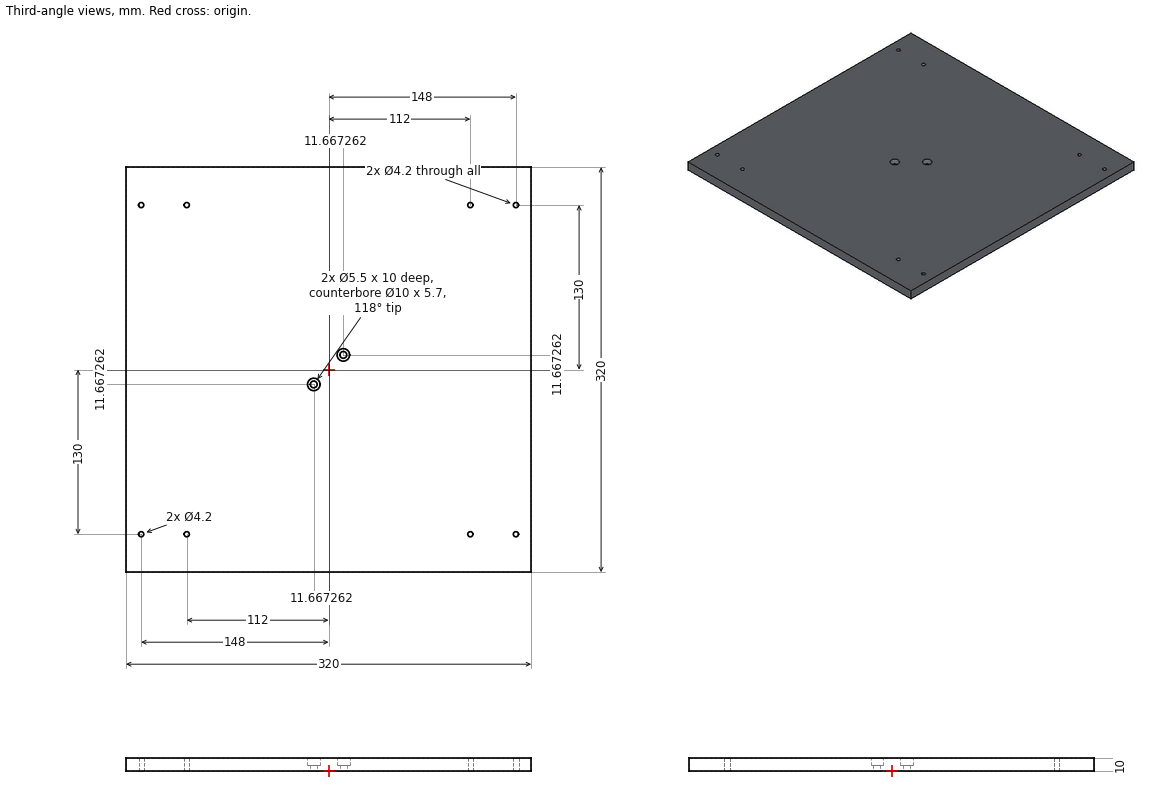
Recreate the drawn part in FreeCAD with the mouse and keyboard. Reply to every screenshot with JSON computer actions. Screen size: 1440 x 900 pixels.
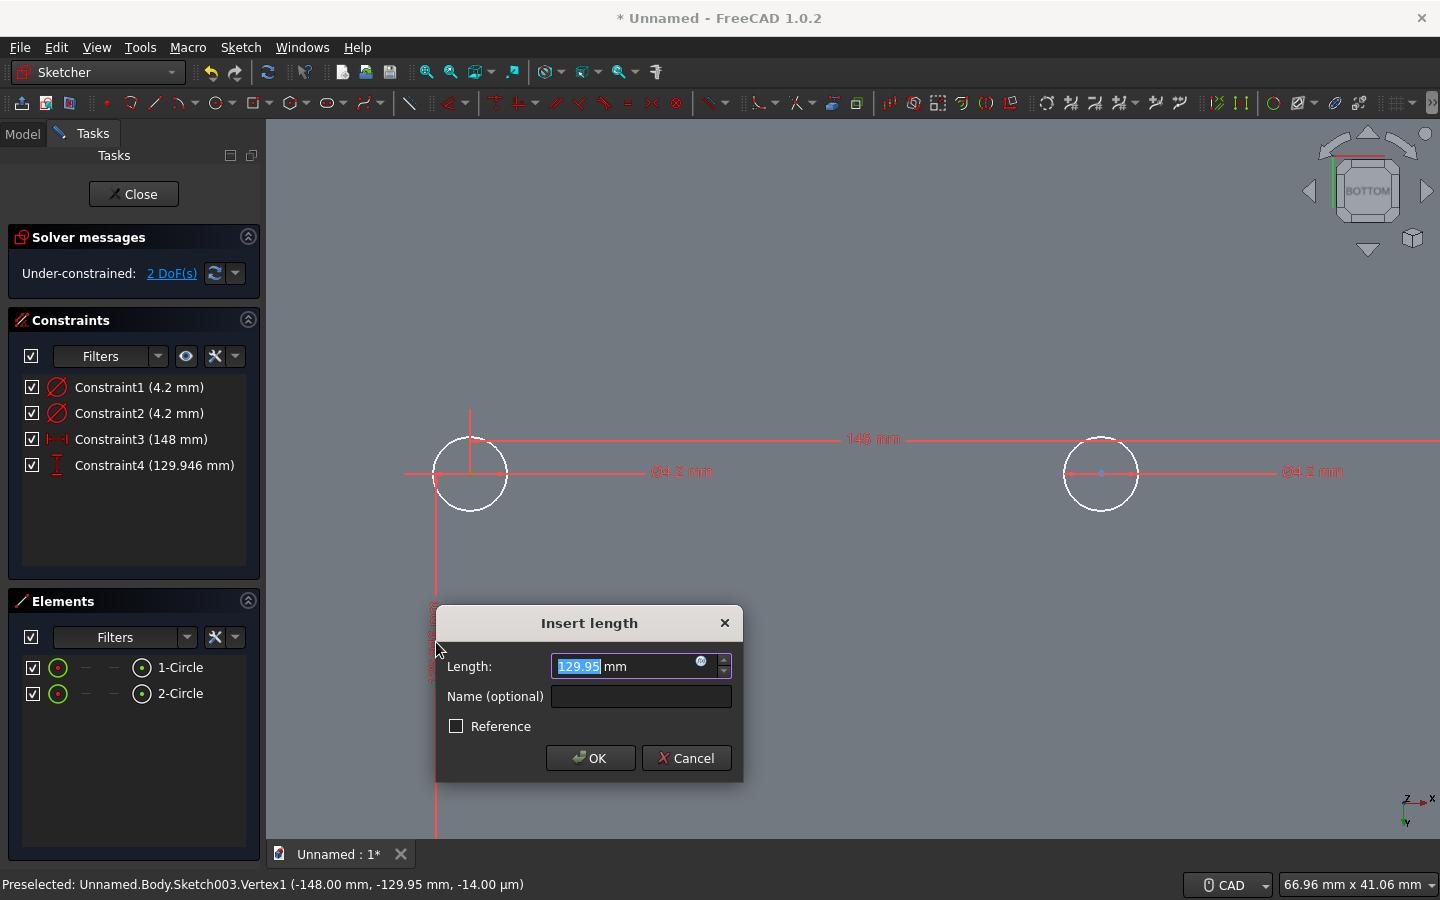
{"action": "type", "text": "130"}
{"action": "key", "text": "Return"}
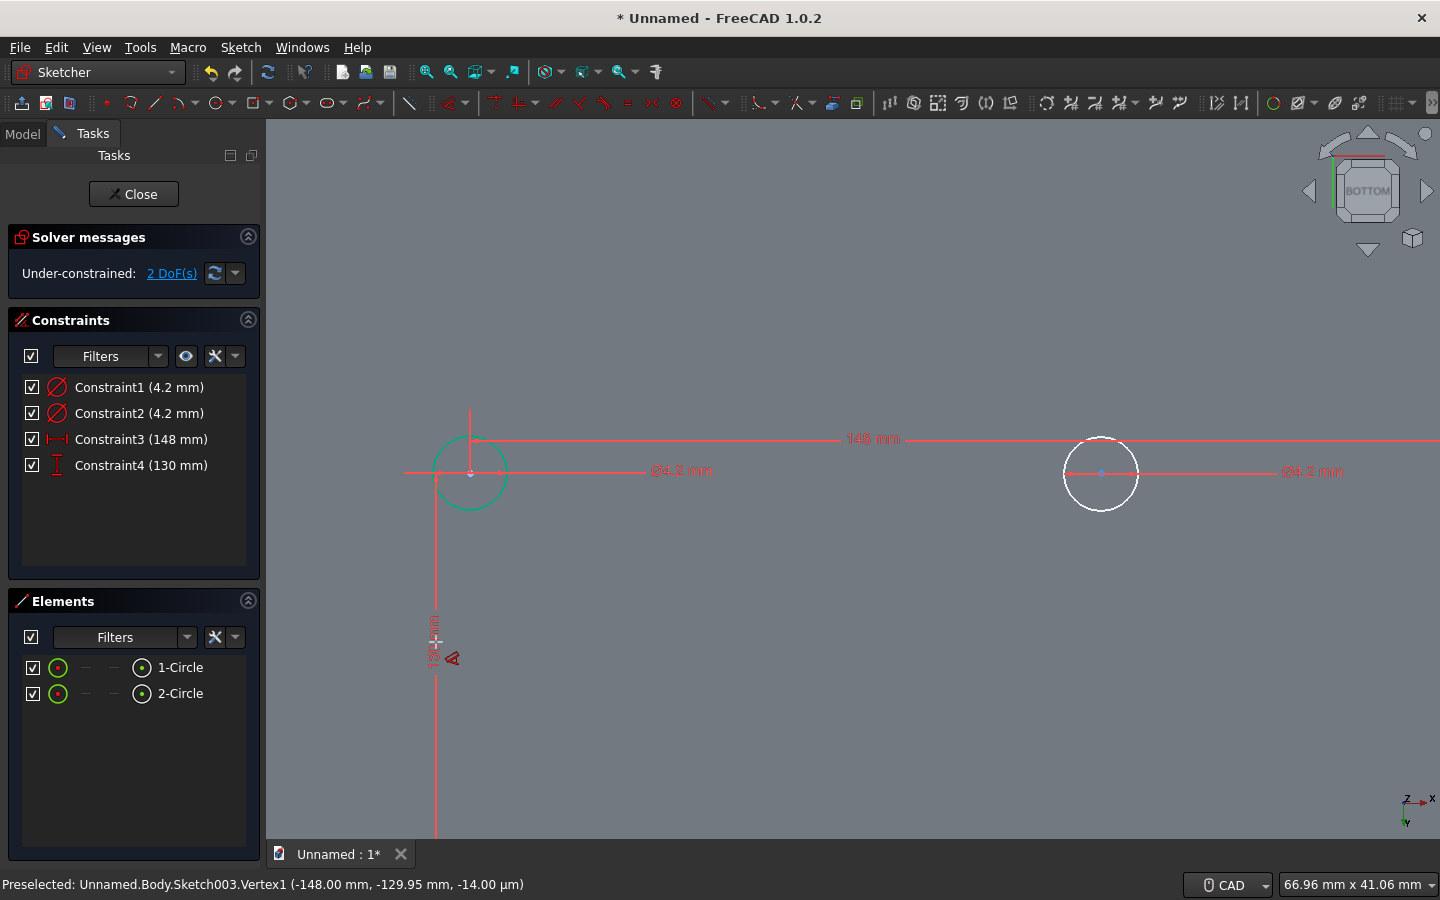
{"action": "left_click", "coordinate": [1101, 474]}
{"action": "left_click", "coordinate": [1188, 440]}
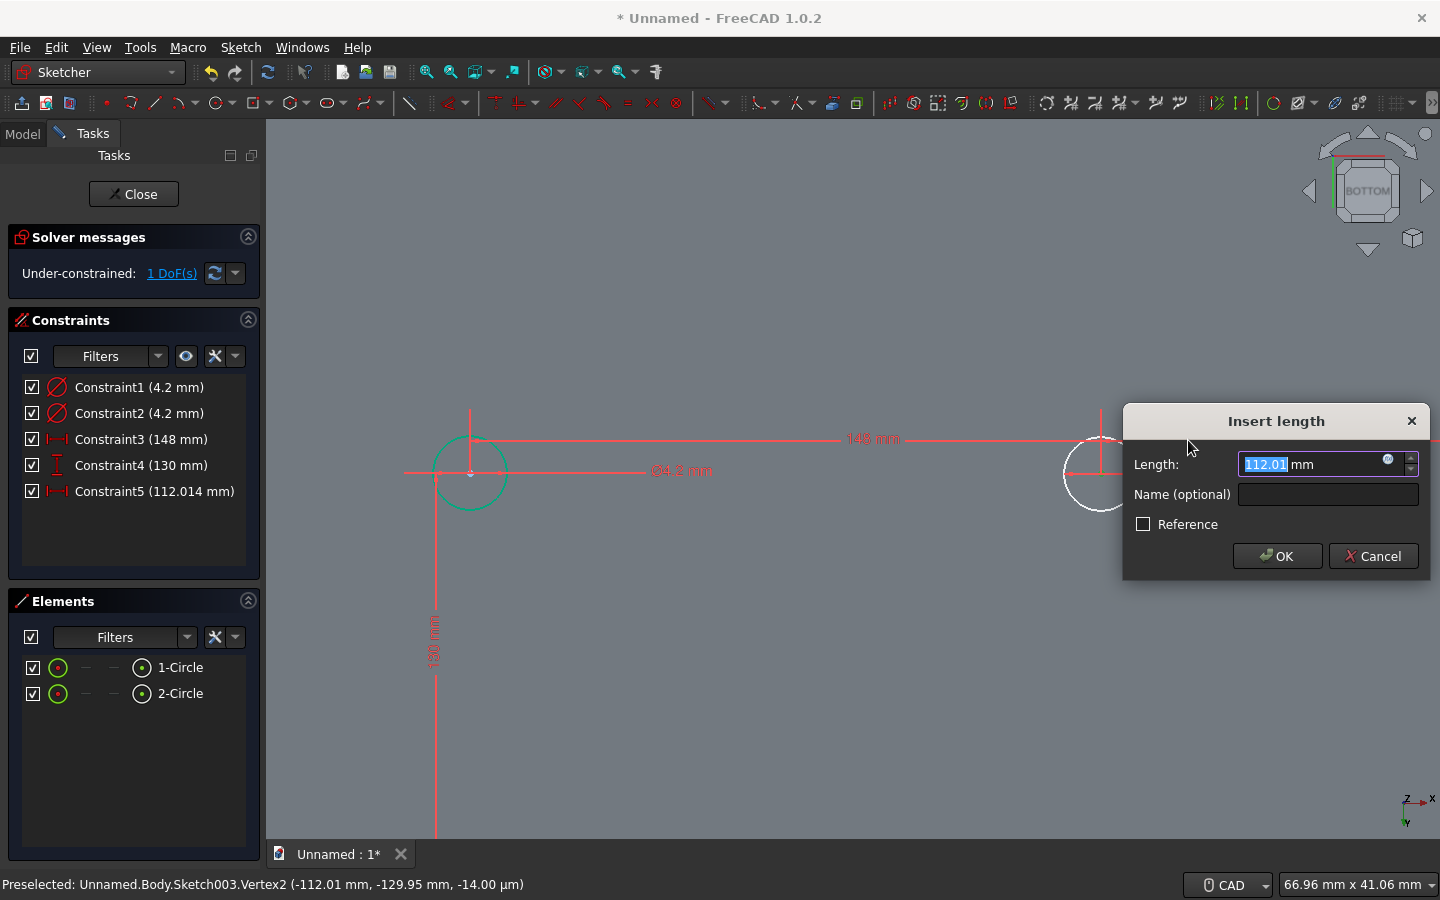
{"action": "type", "text": "112"}
{"action": "key", "text": "Return"}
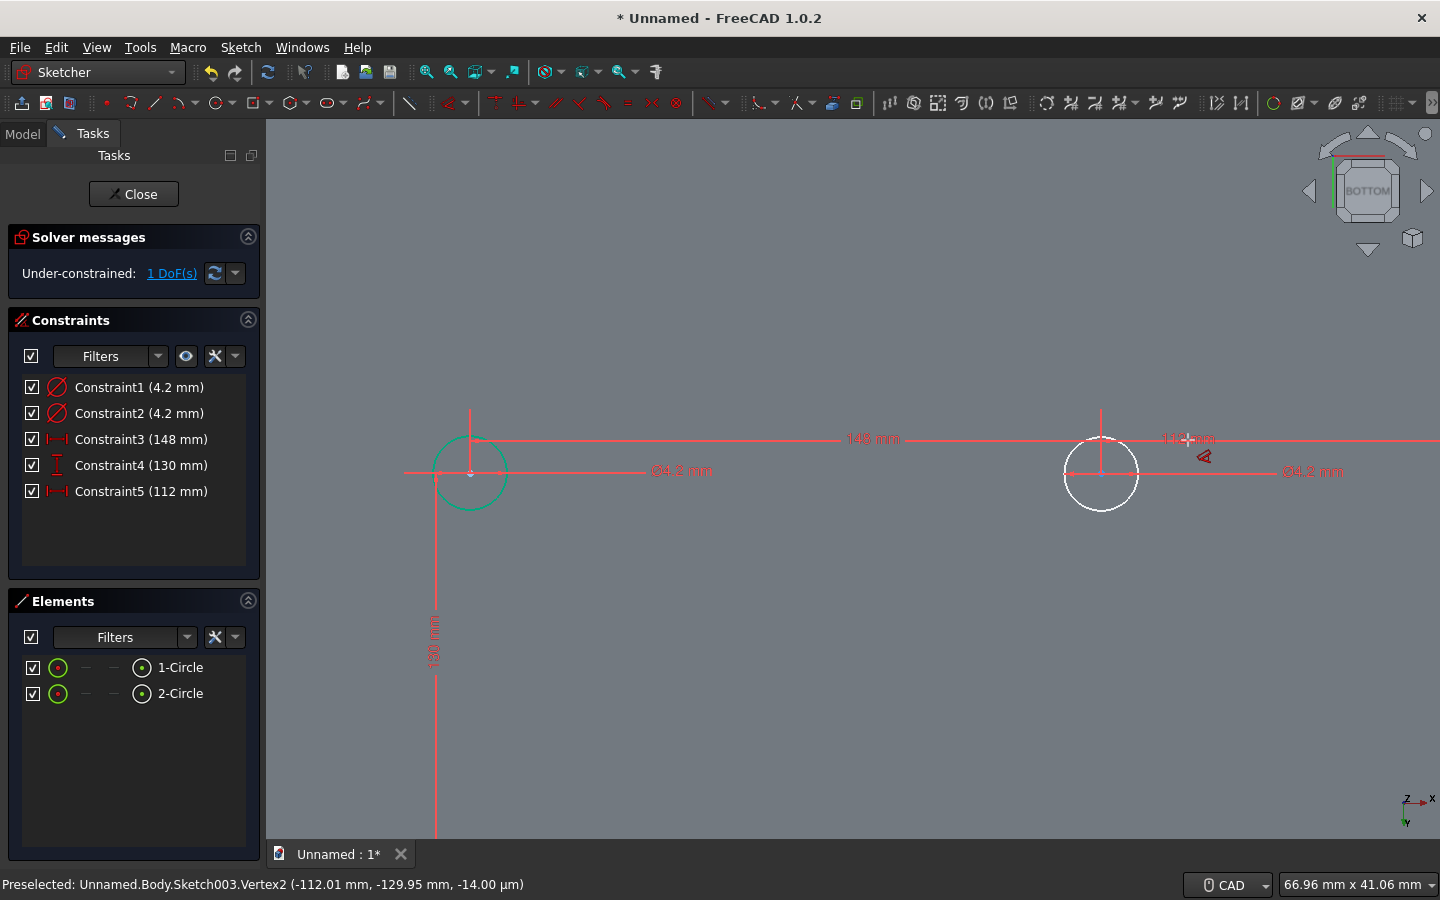
{"action": "left_click", "coordinate": [1101, 474]}
{"action": "left_click", "coordinate": [1067, 642]}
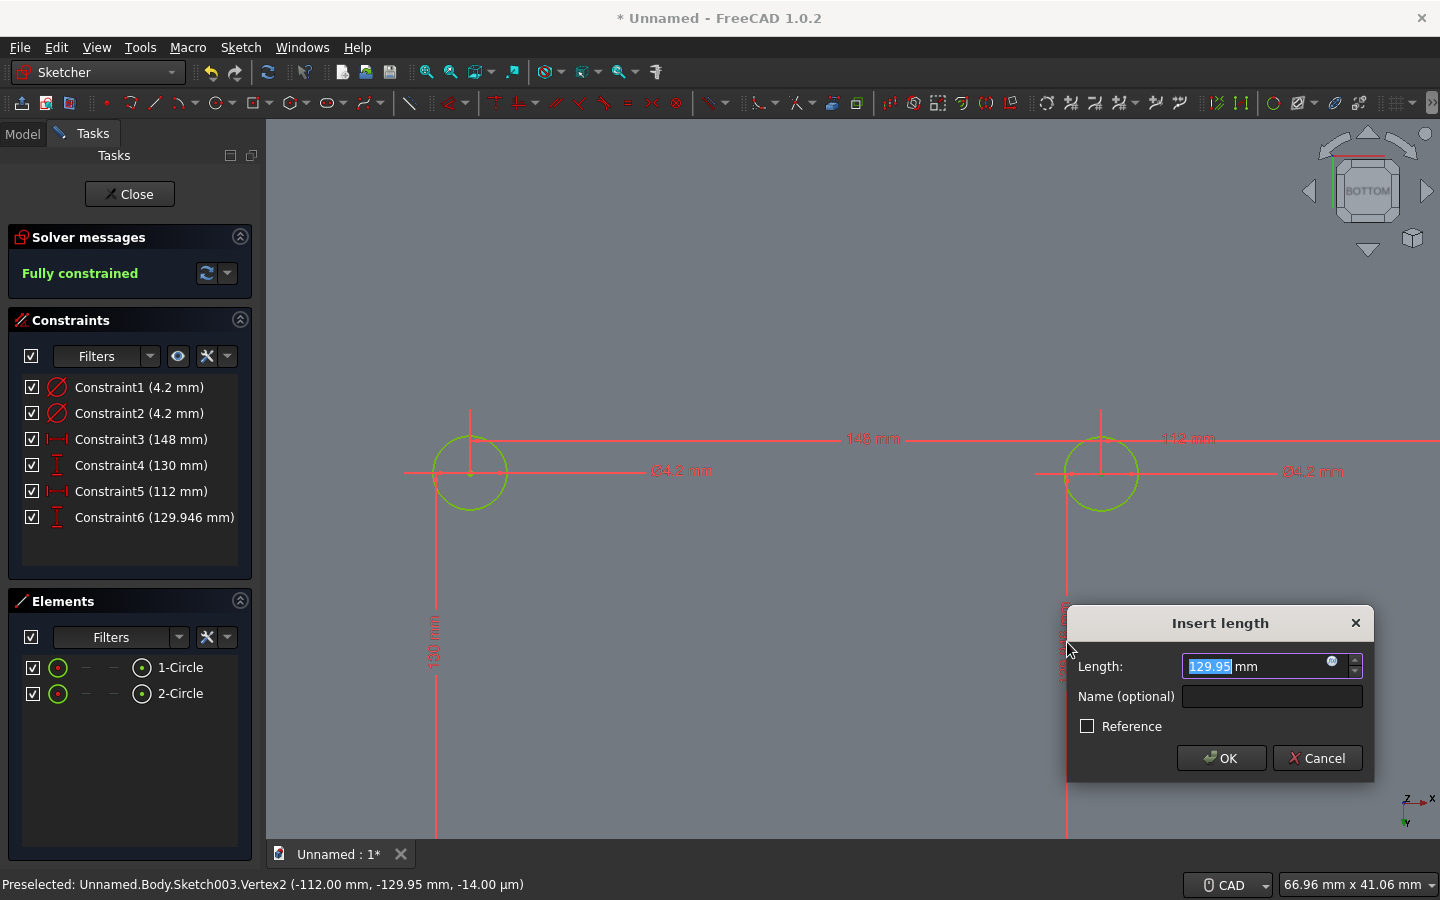
{"action": "type", "text": "130"}
{"action": "key", "text": "Return"}
{"action": "key", "text": "Escape"}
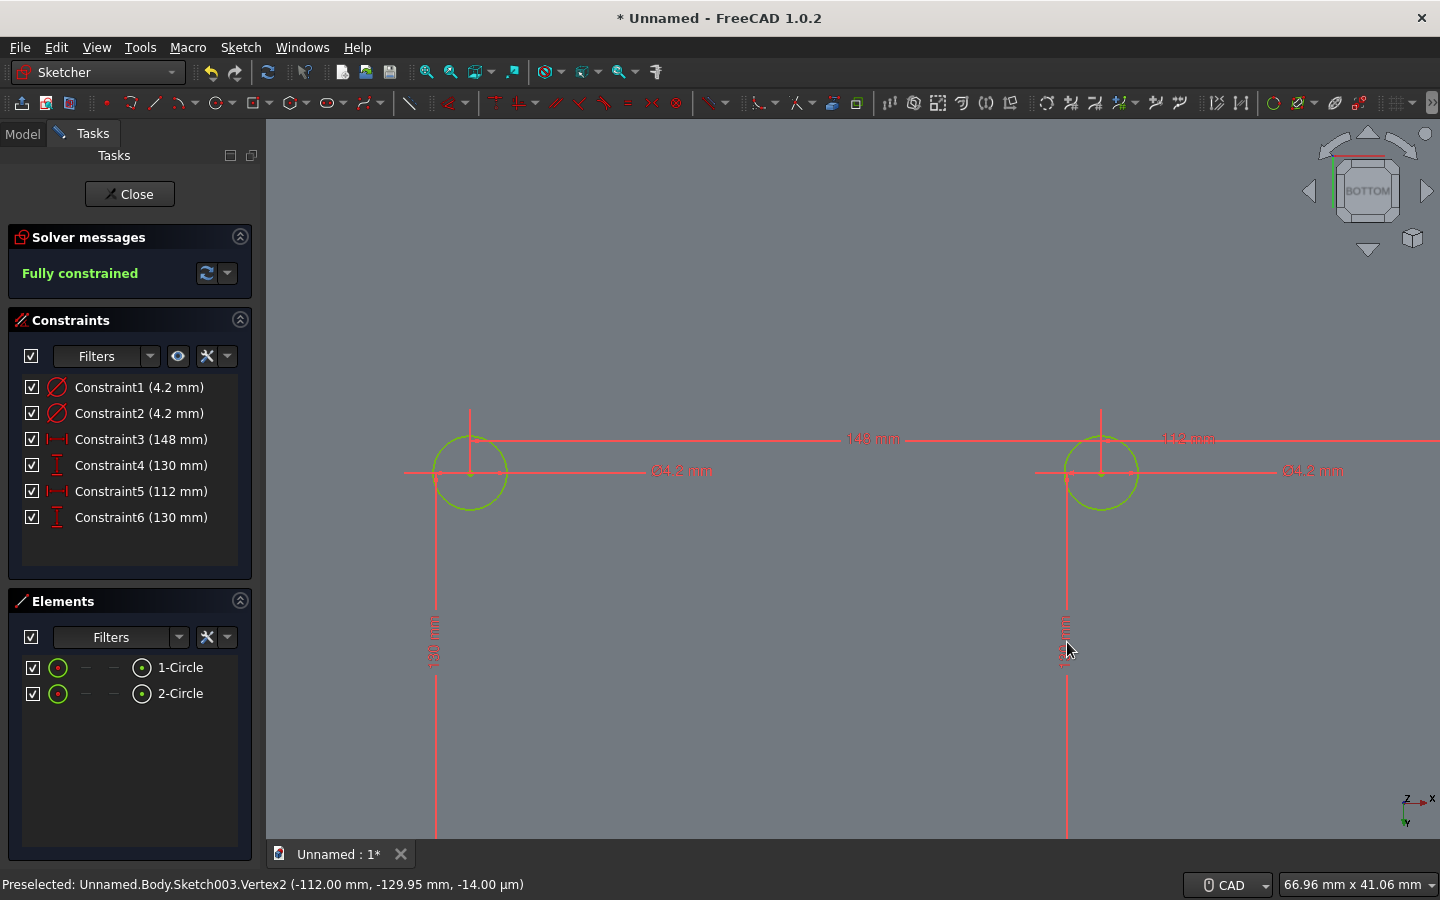
{"action": "left_click", "coordinate": [130, 194]}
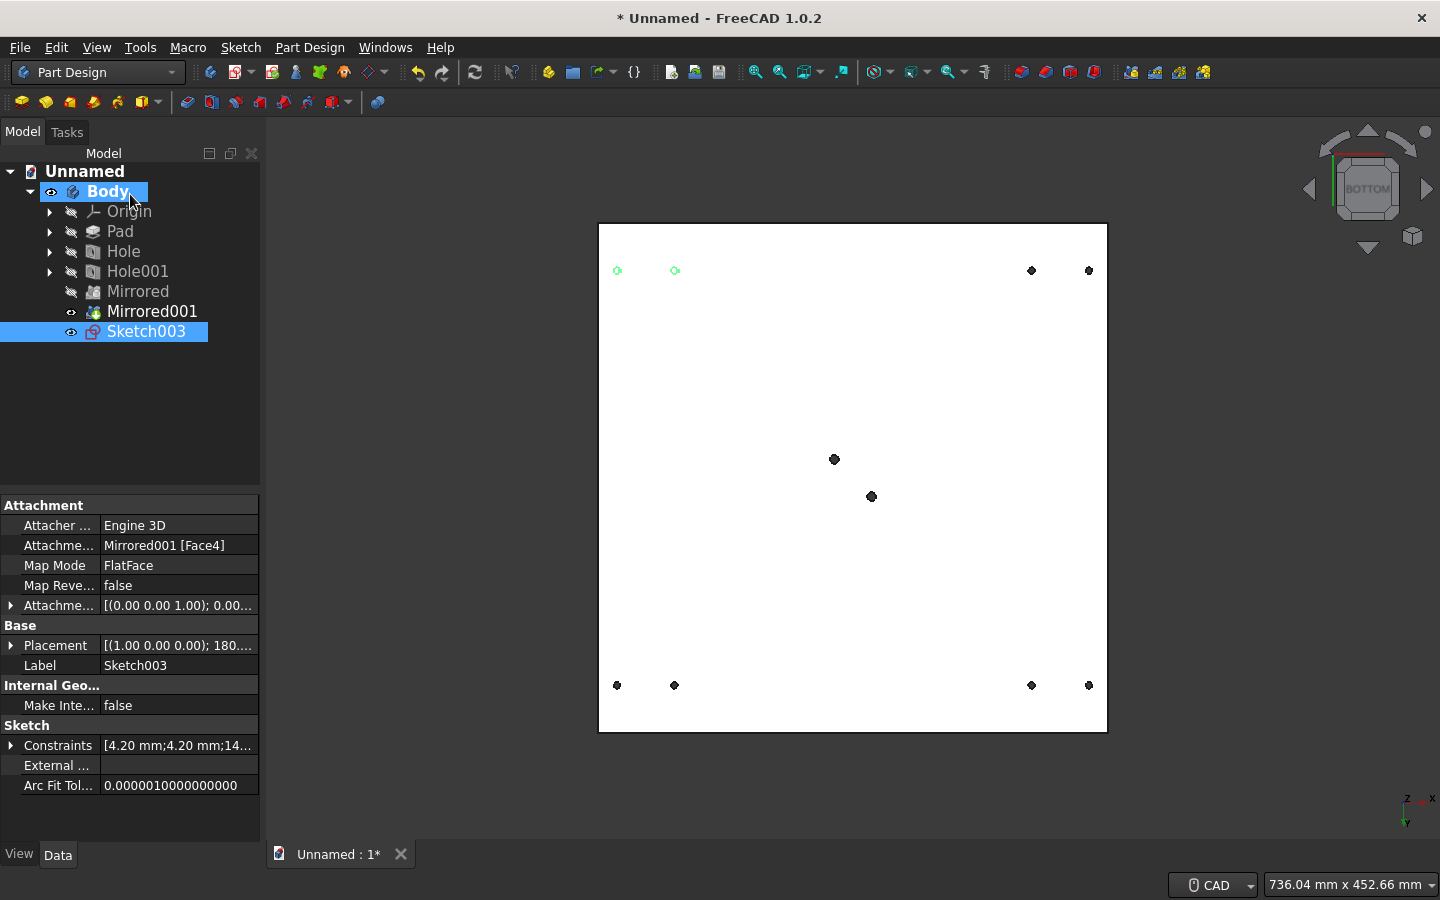
{"action": "left_click", "coordinate": [188, 102]}